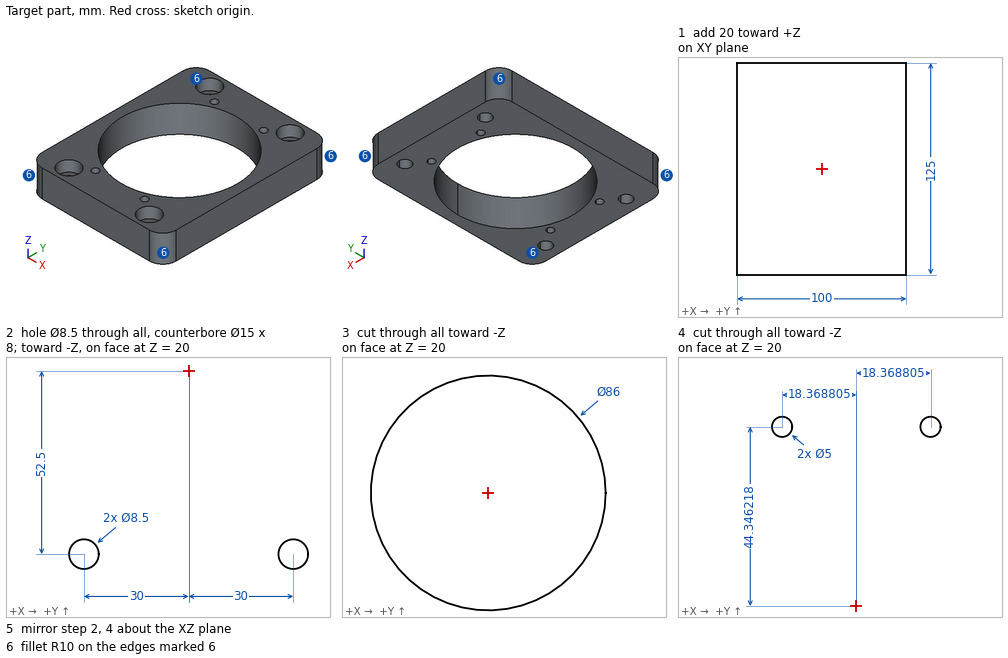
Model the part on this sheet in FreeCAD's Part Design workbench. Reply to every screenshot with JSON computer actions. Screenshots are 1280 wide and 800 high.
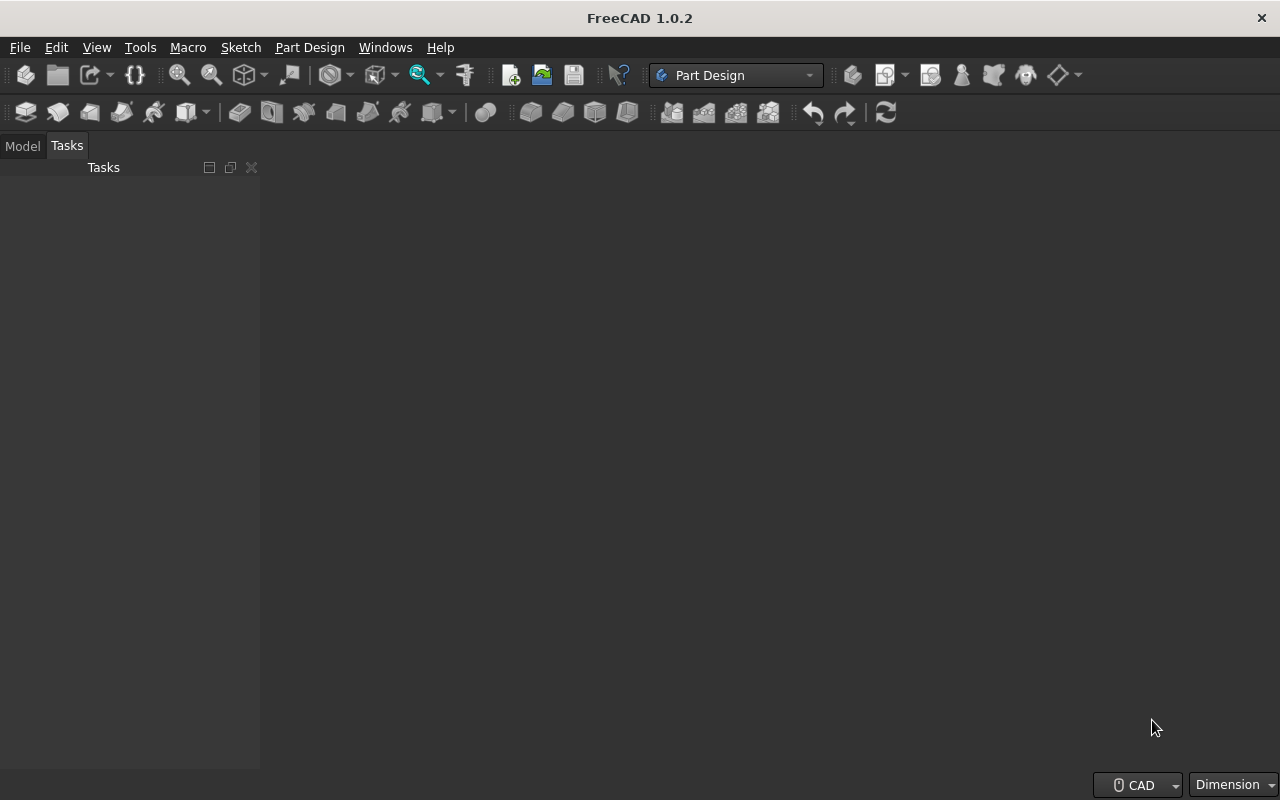
{"action": "left_click", "coordinate": [510, 76]}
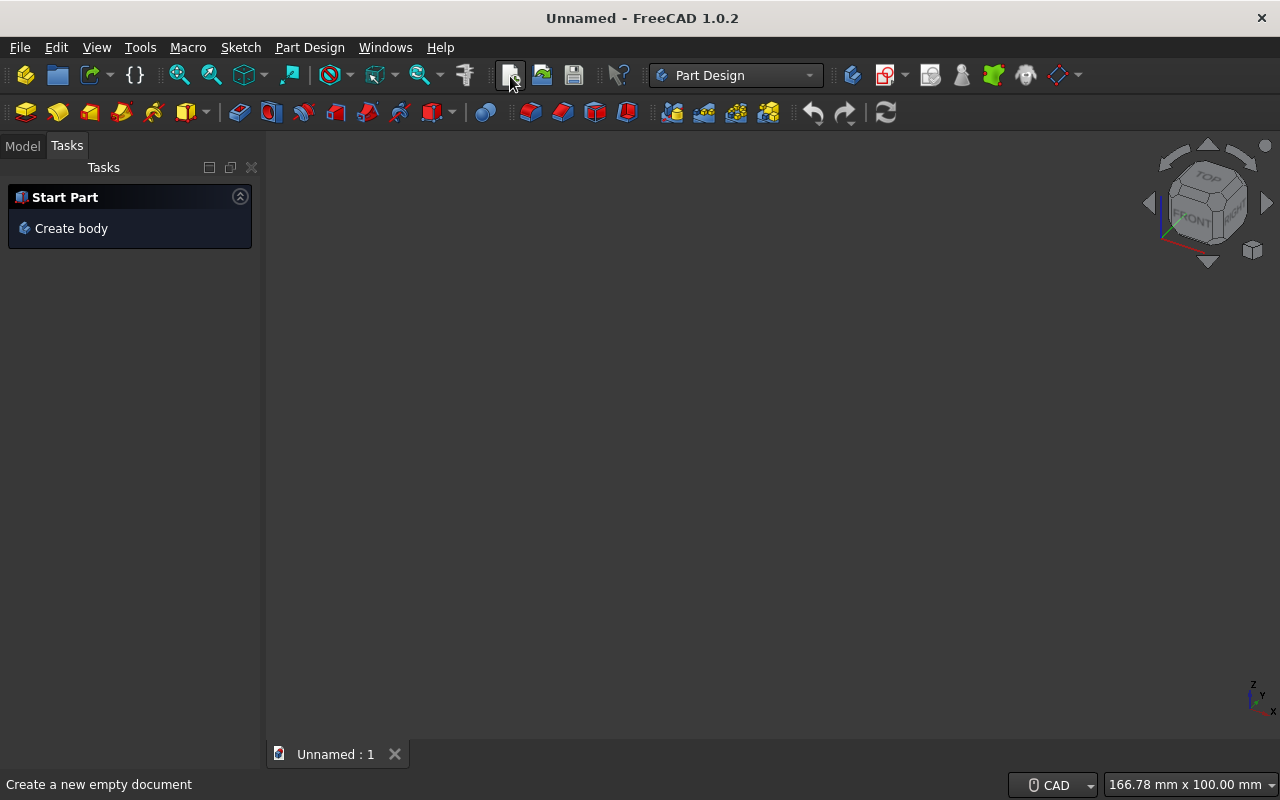
{"action": "left_click", "coordinate": [886, 76]}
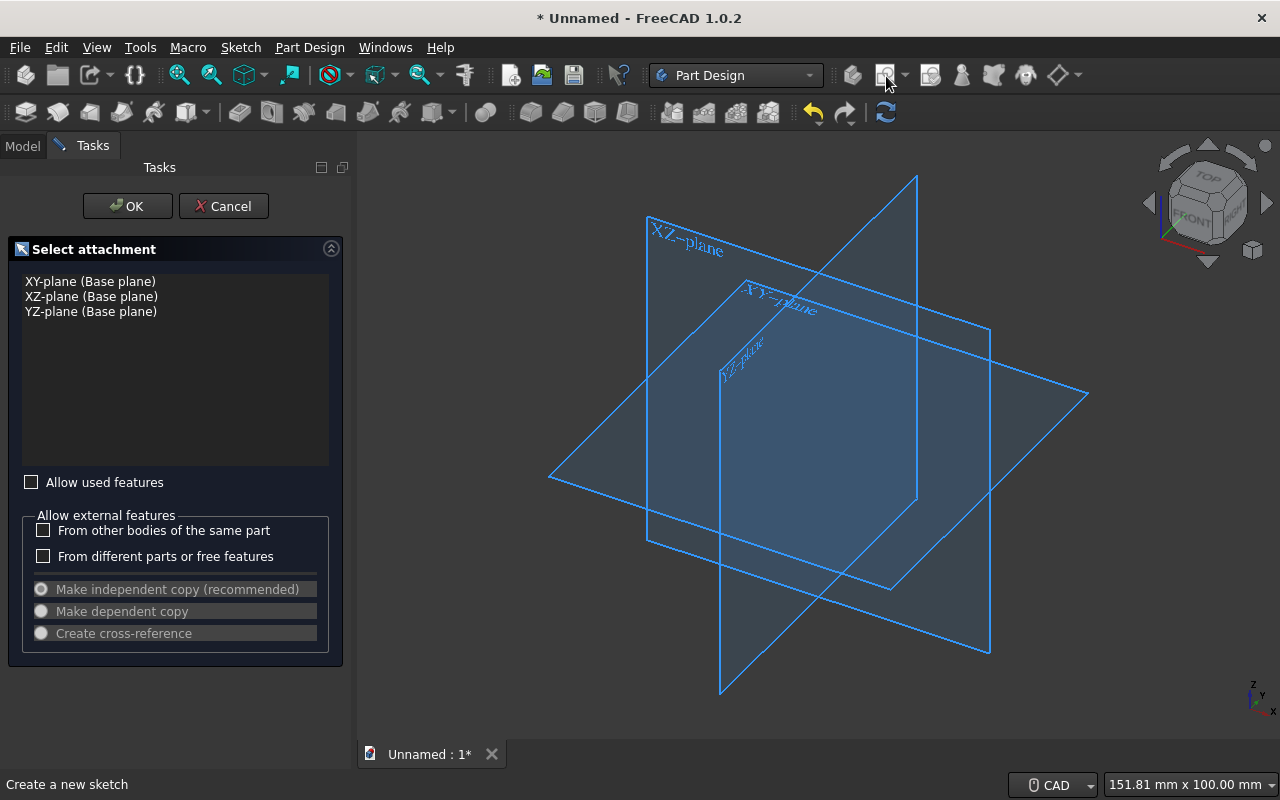
{"action": "left_click", "coordinate": [82, 282]}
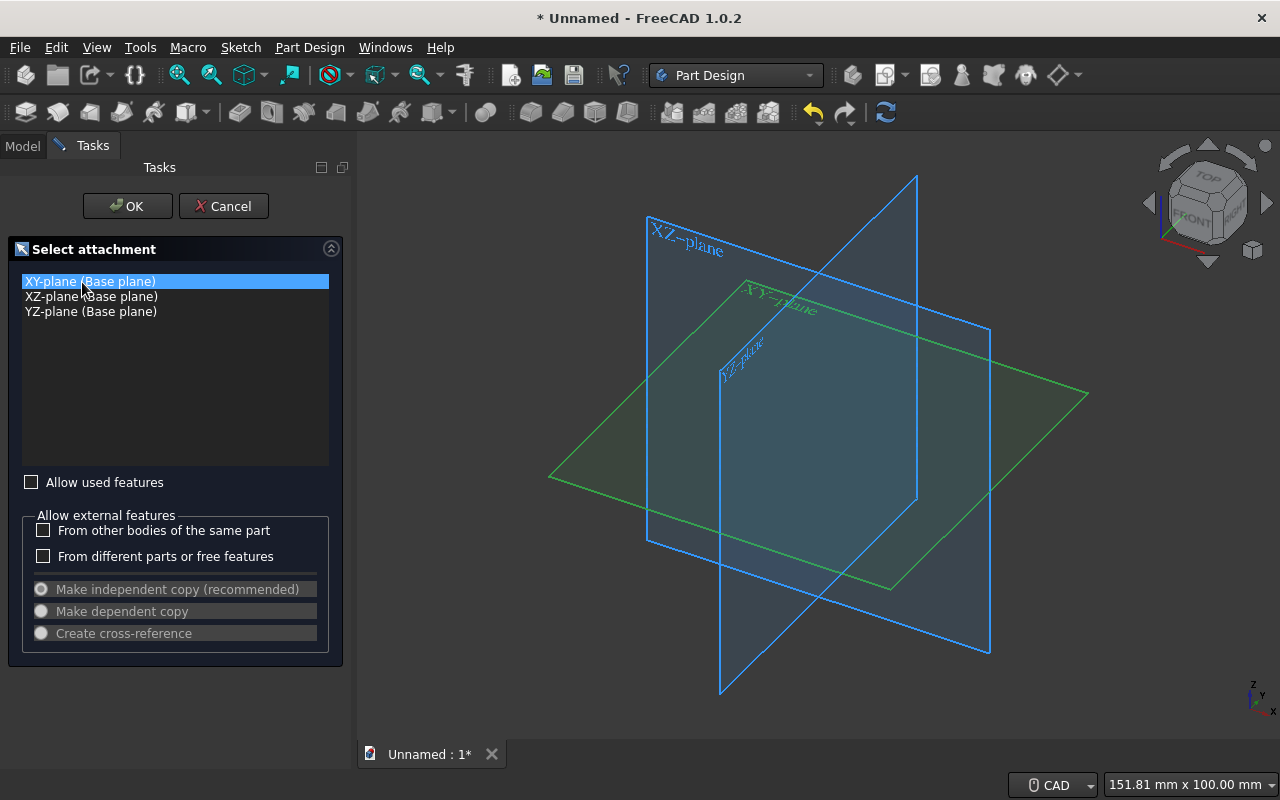
{"action": "left_click", "coordinate": [128, 206]}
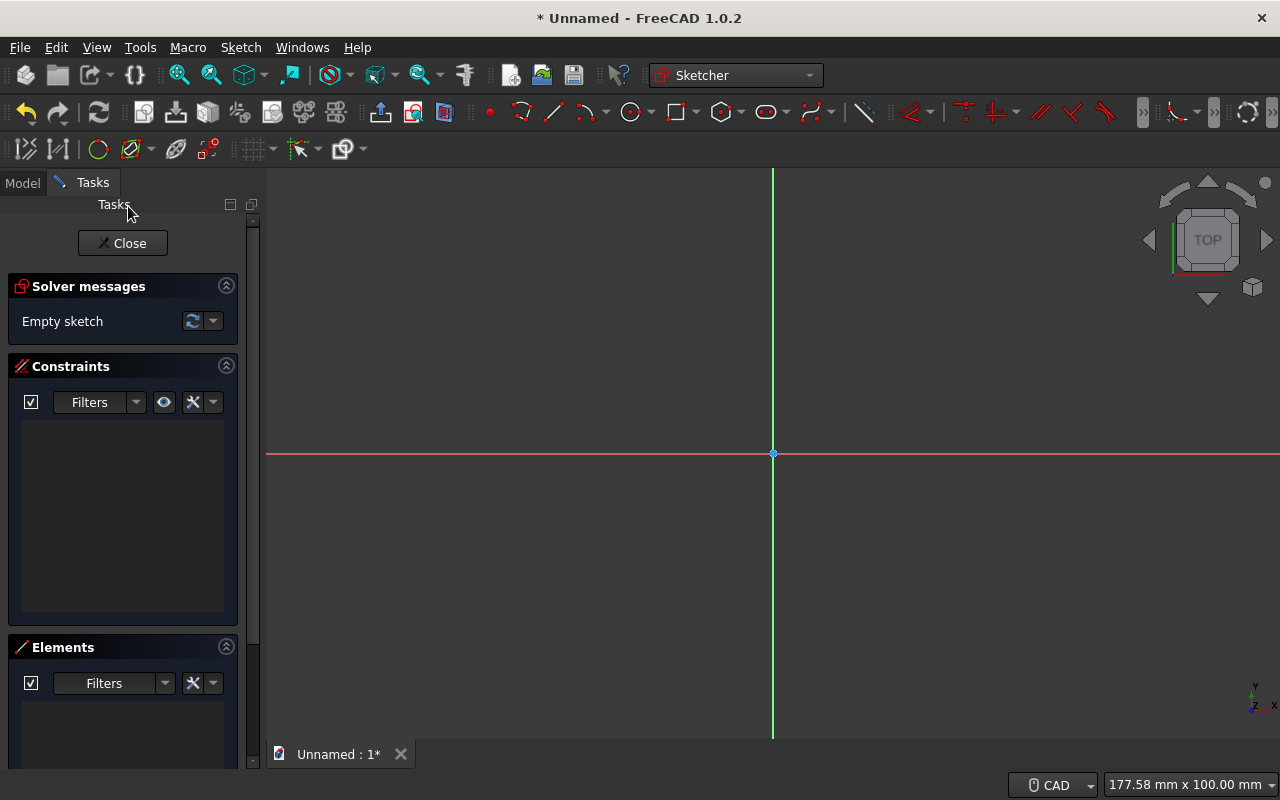
{"action": "scroll", "coordinate": [621, 454], "scroll_direction": "down", "scroll_amount": 3}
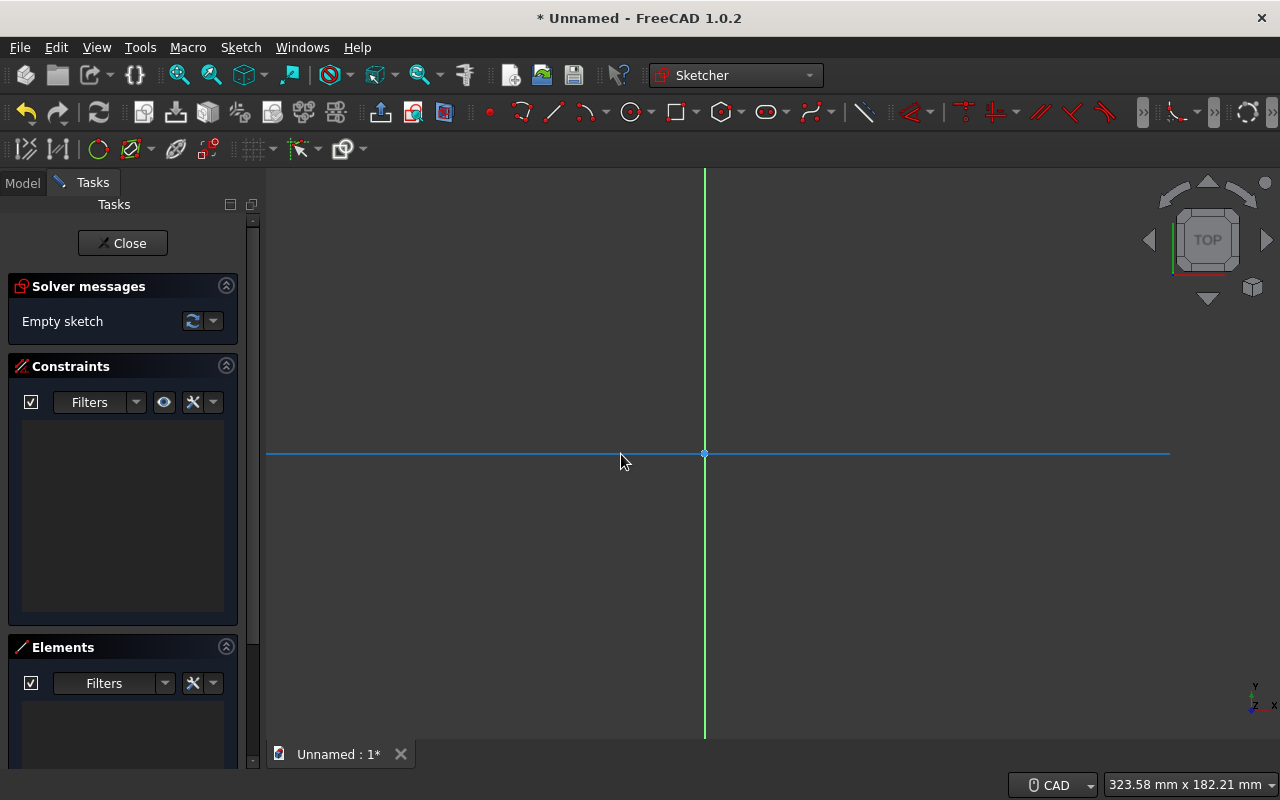
{"action": "left_click", "coordinate": [698, 112]}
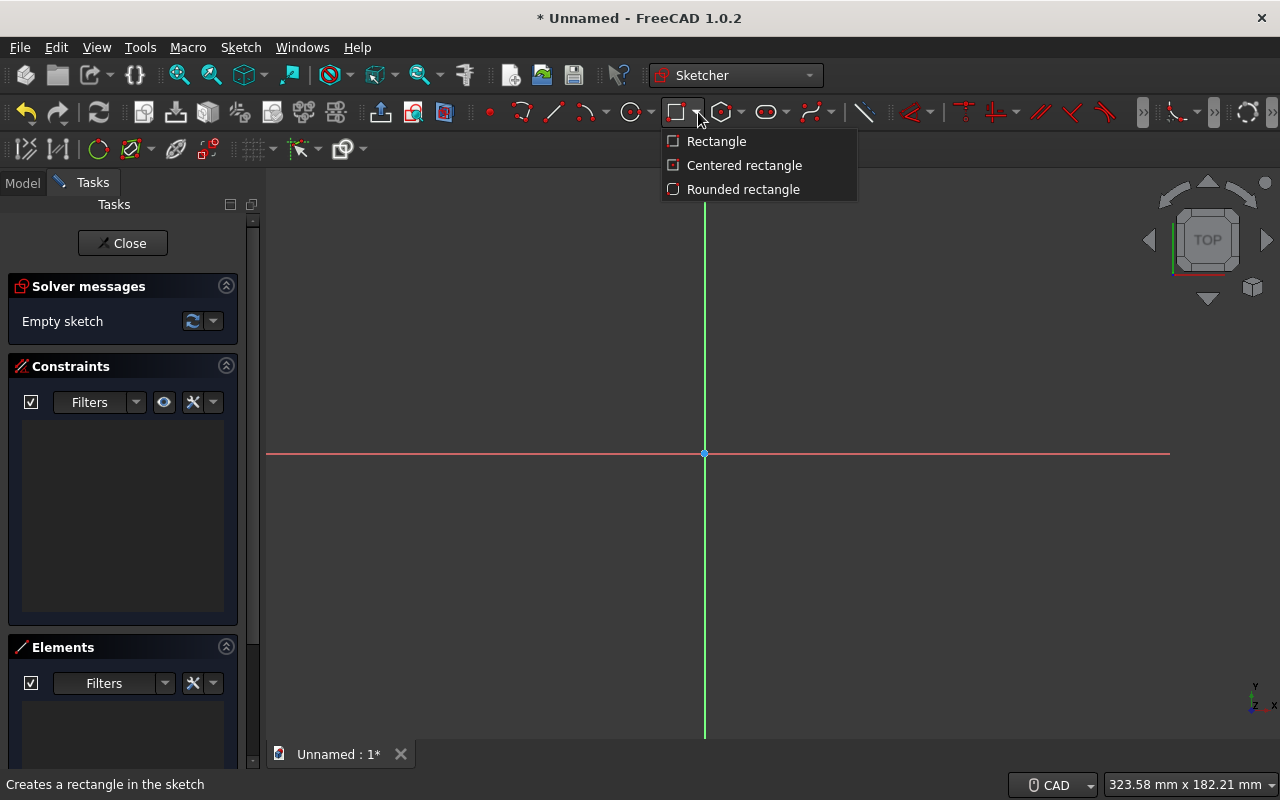
{"action": "left_click", "coordinate": [760, 165]}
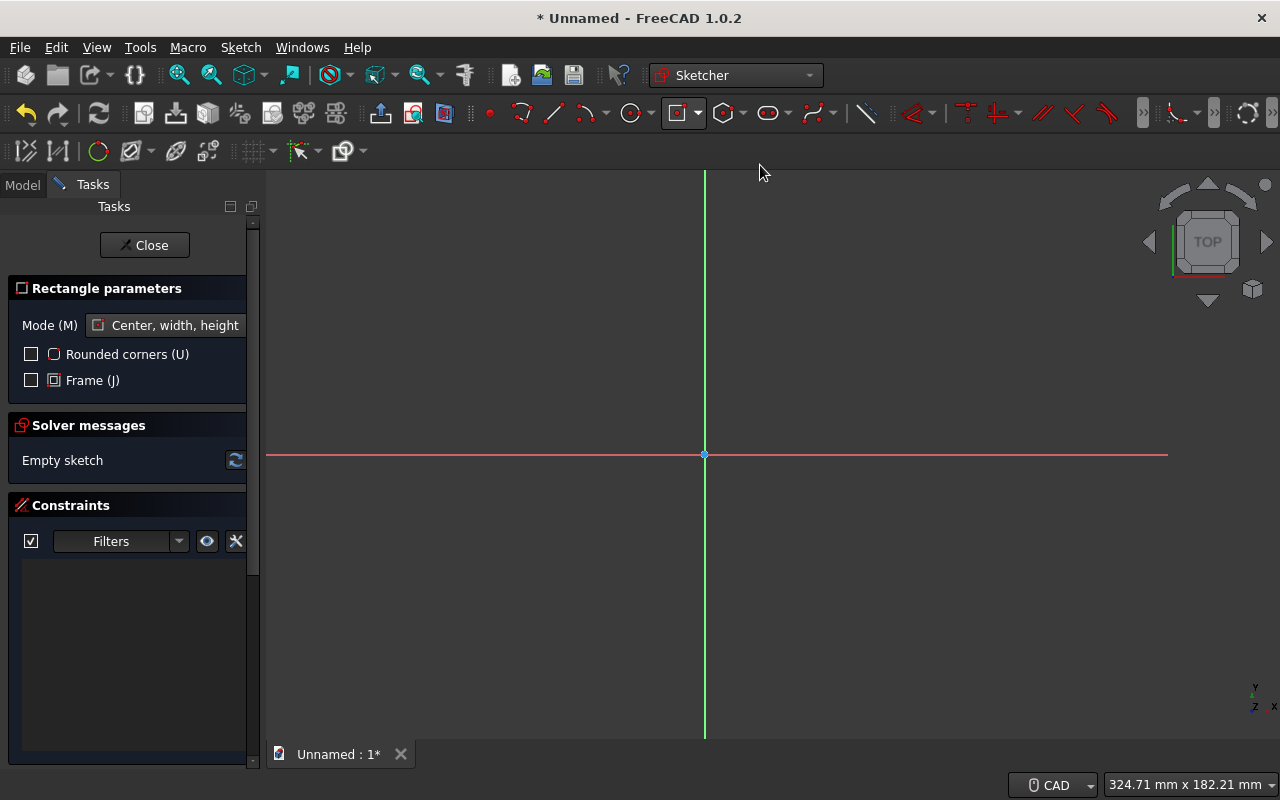
{"action": "left_click", "coordinate": [705, 455]}
{"action": "mouse_move", "coordinate": [861, 260]}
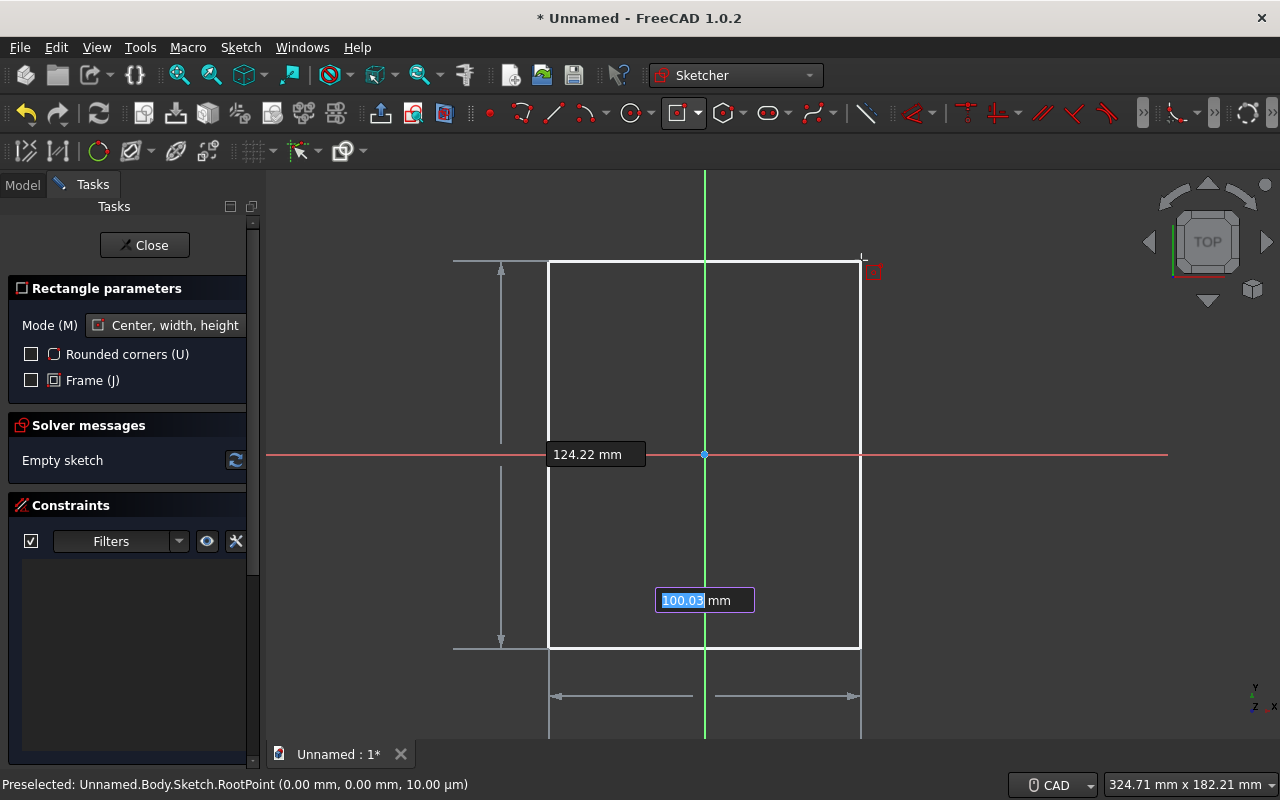
{"action": "type", "text": "100"}
{"action": "key", "text": "Tab"}
{"action": "type", "text": "125"}
{"action": "key", "text": "Return"}
{"action": "key", "text": "Escape"}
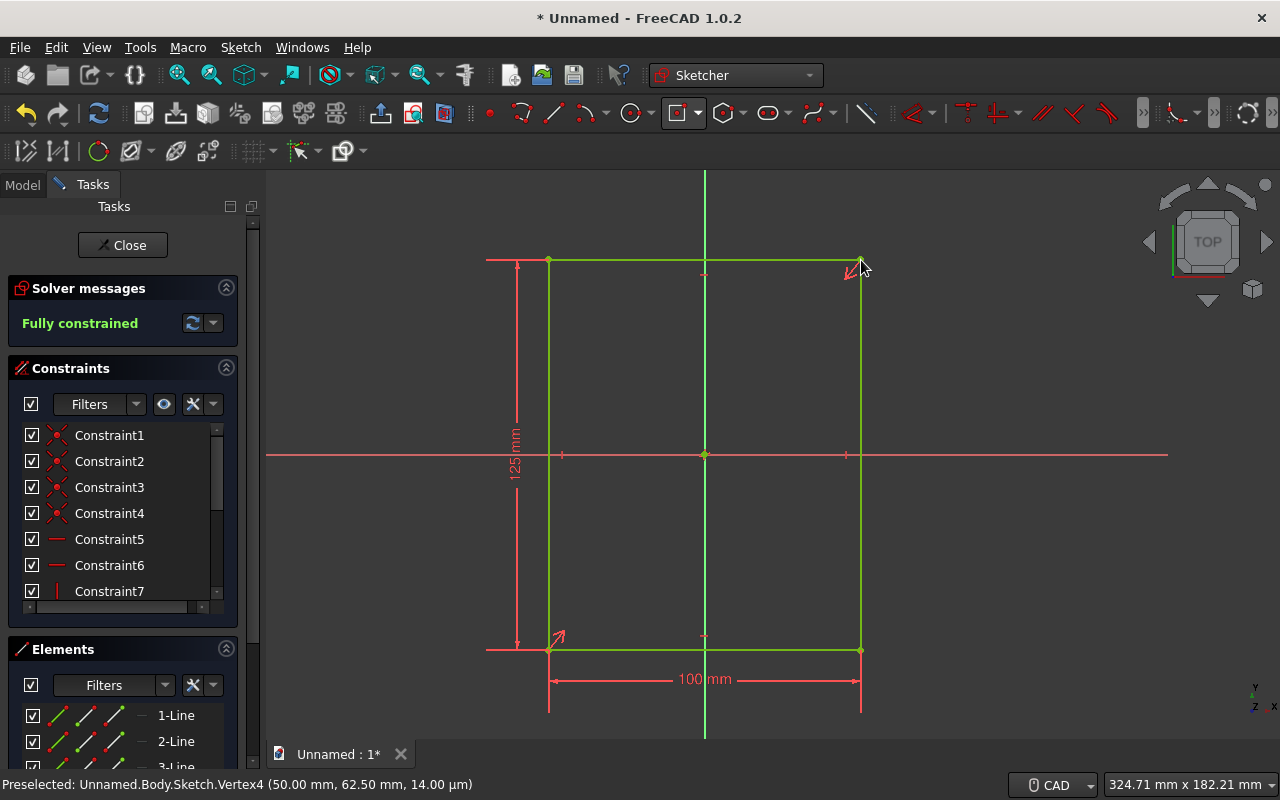
{"action": "left_click", "coordinate": [123, 245]}